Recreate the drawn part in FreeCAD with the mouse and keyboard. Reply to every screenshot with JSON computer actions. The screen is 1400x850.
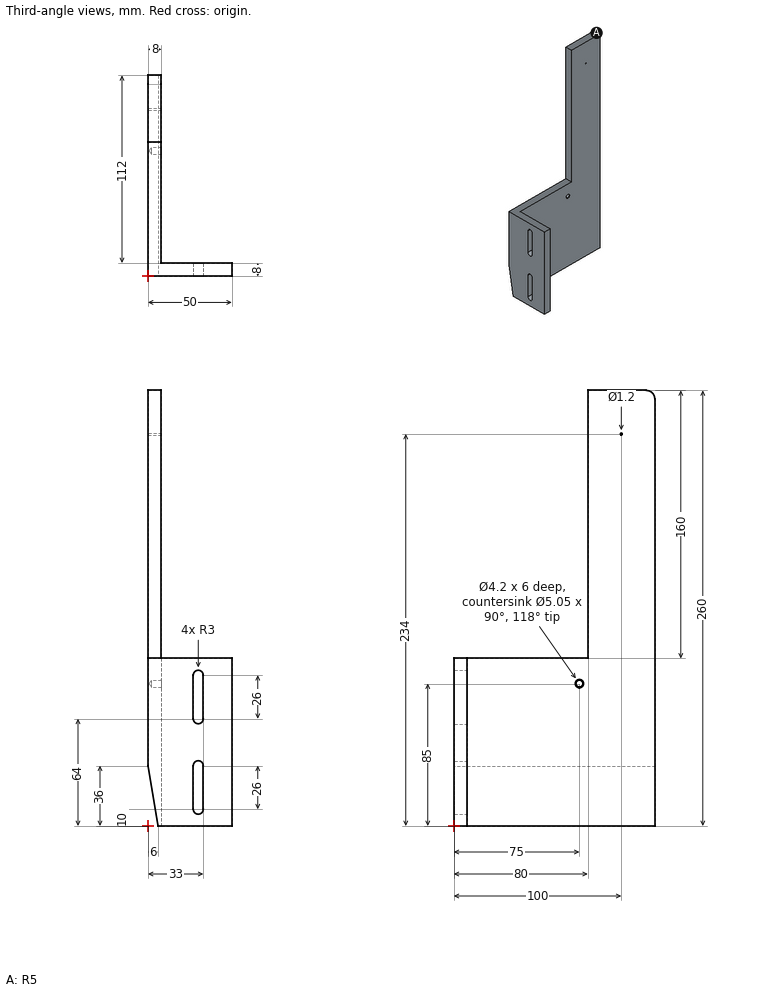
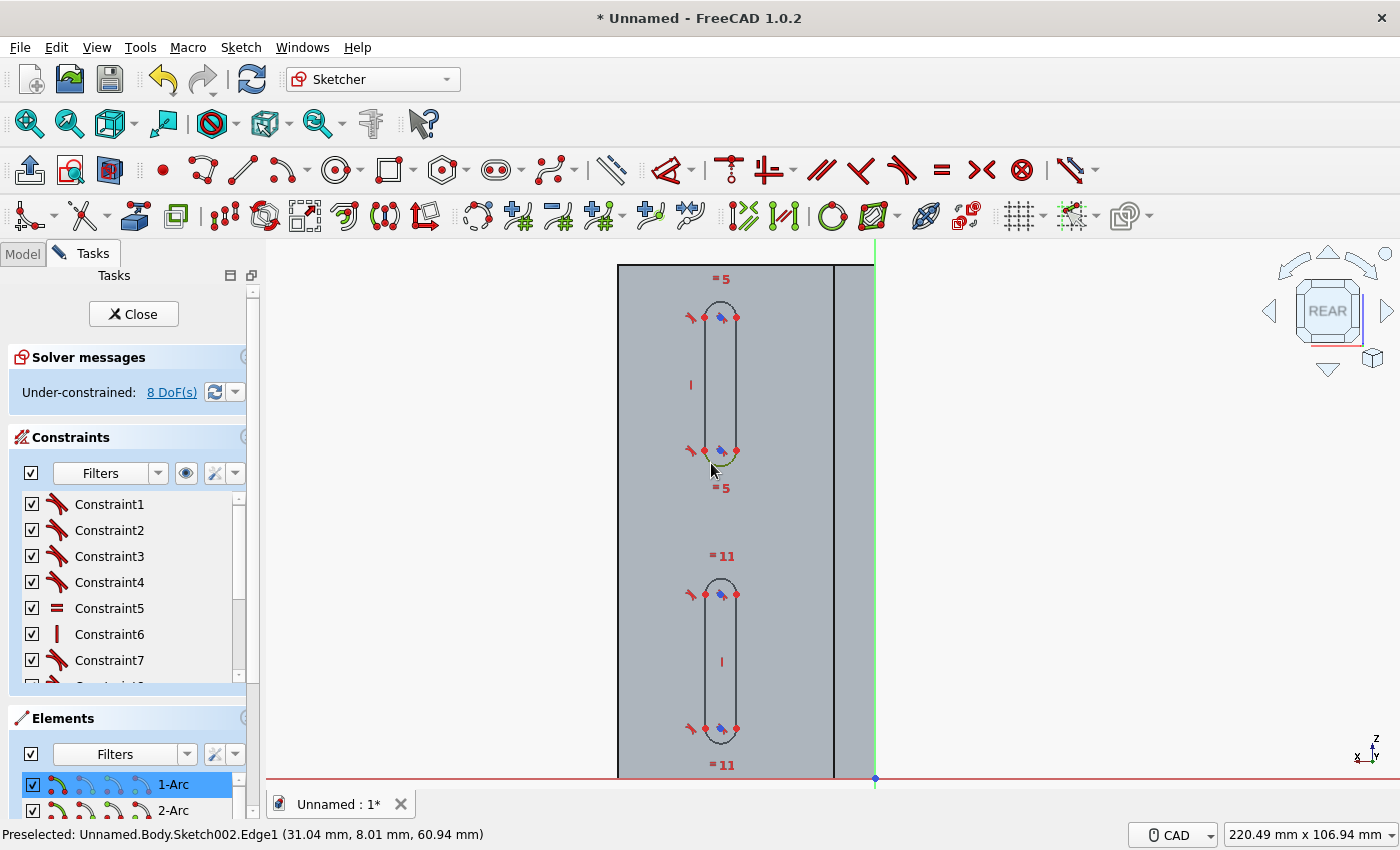
{"action": "left_click", "coordinate": [712, 741]}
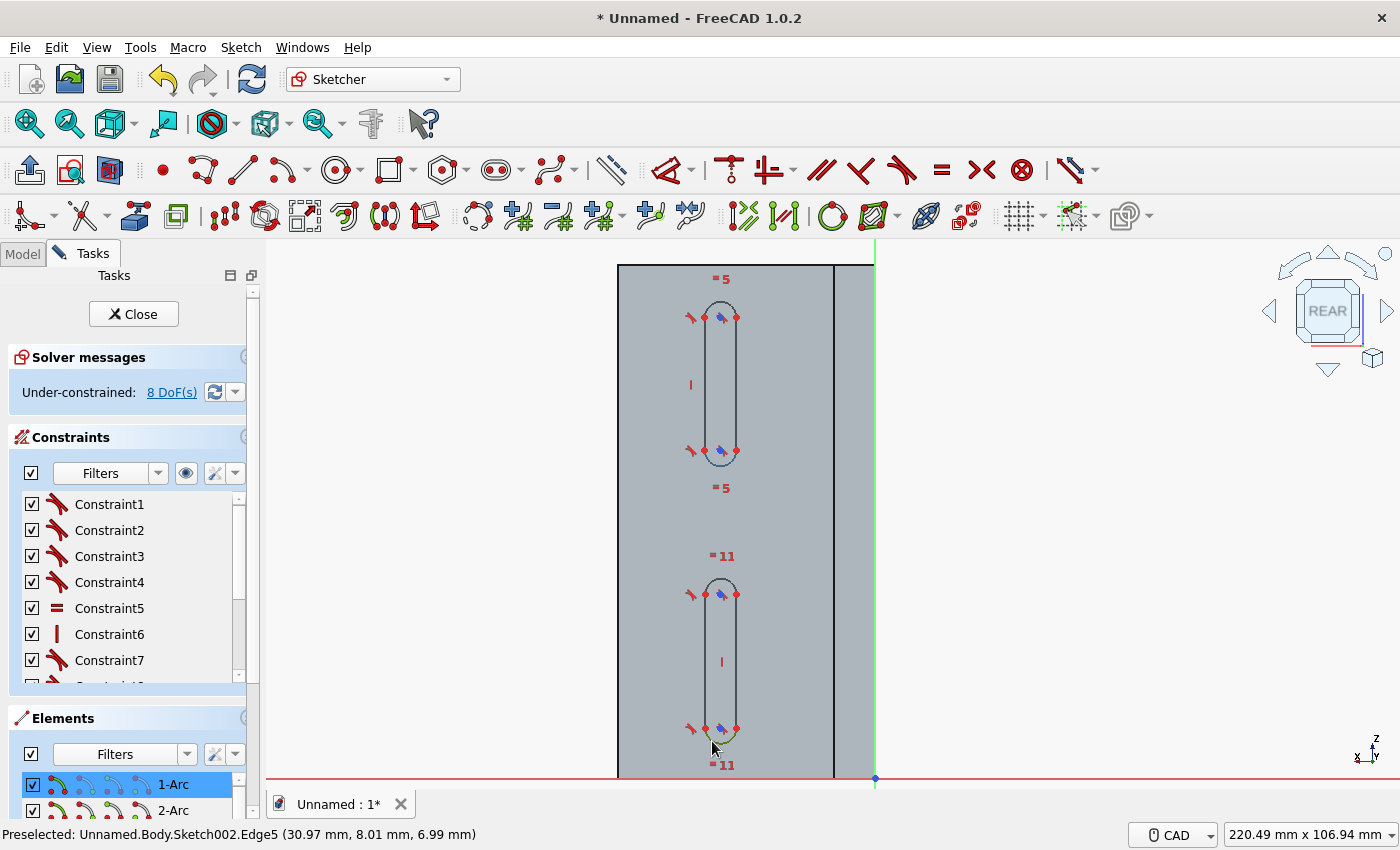
{"action": "left_click", "coordinate": [942, 170]}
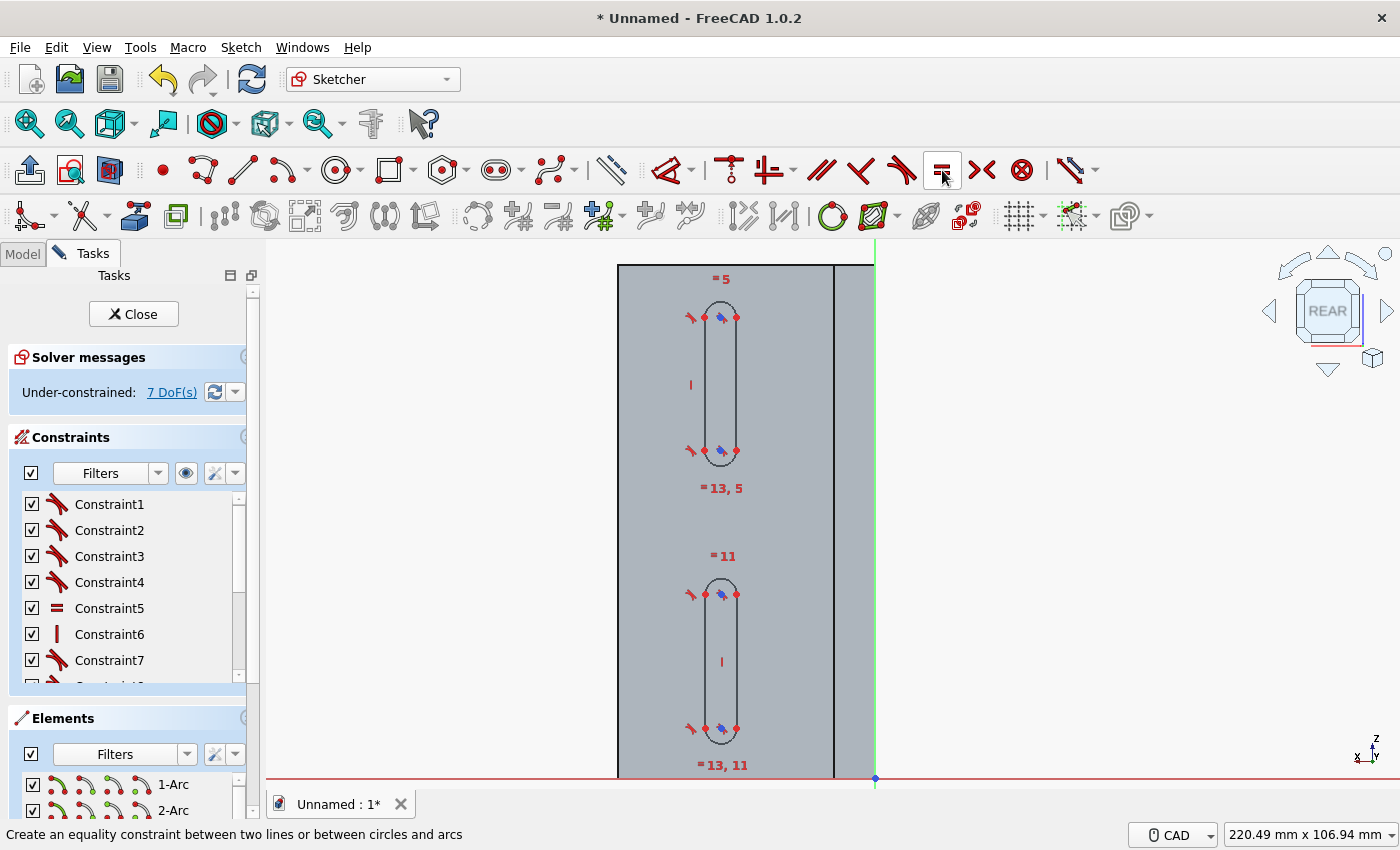
{"action": "left_click", "coordinate": [666, 170]}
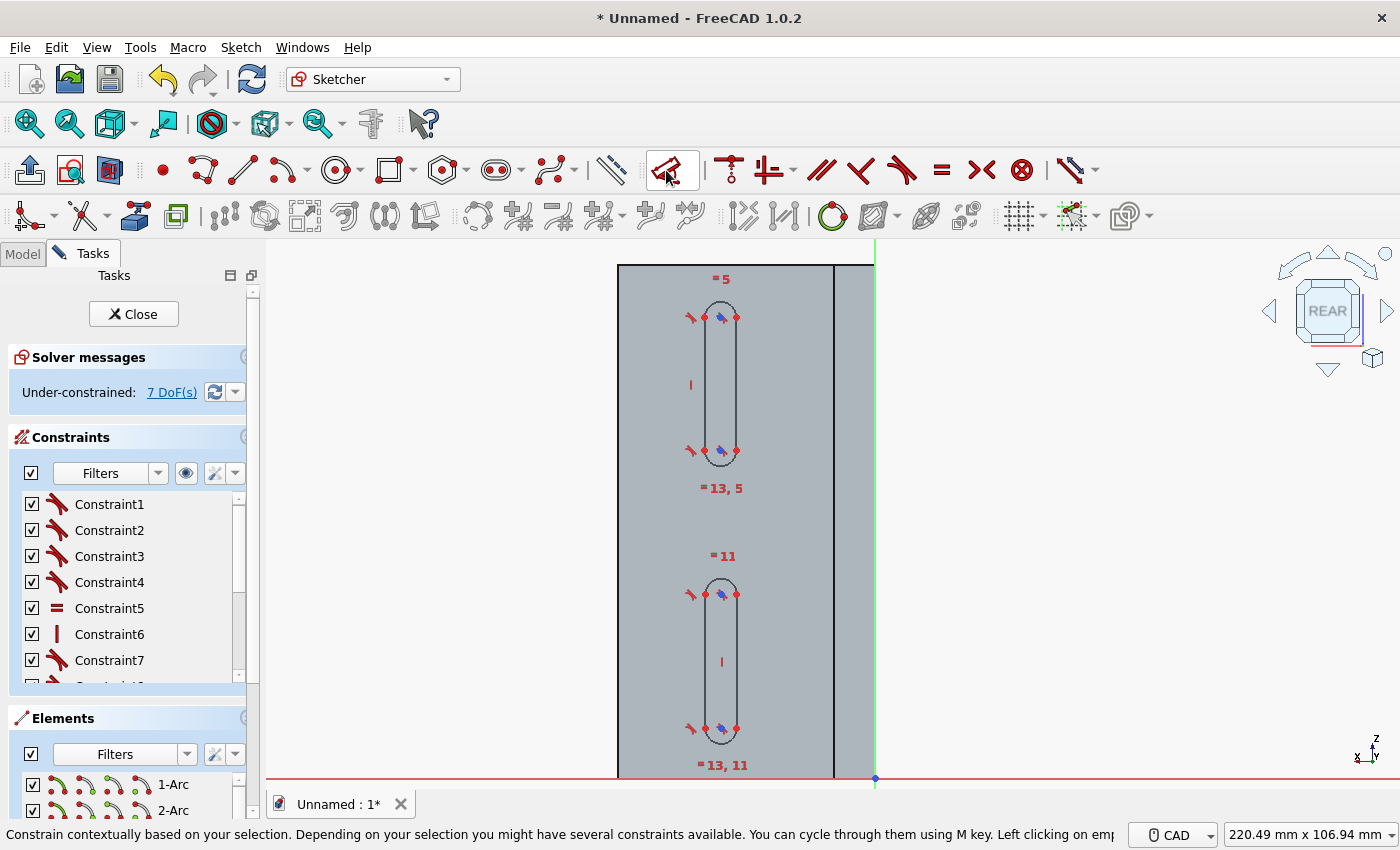
{"action": "scroll", "coordinate": [711, 463], "scroll_direction": "up", "scroll_amount": 5}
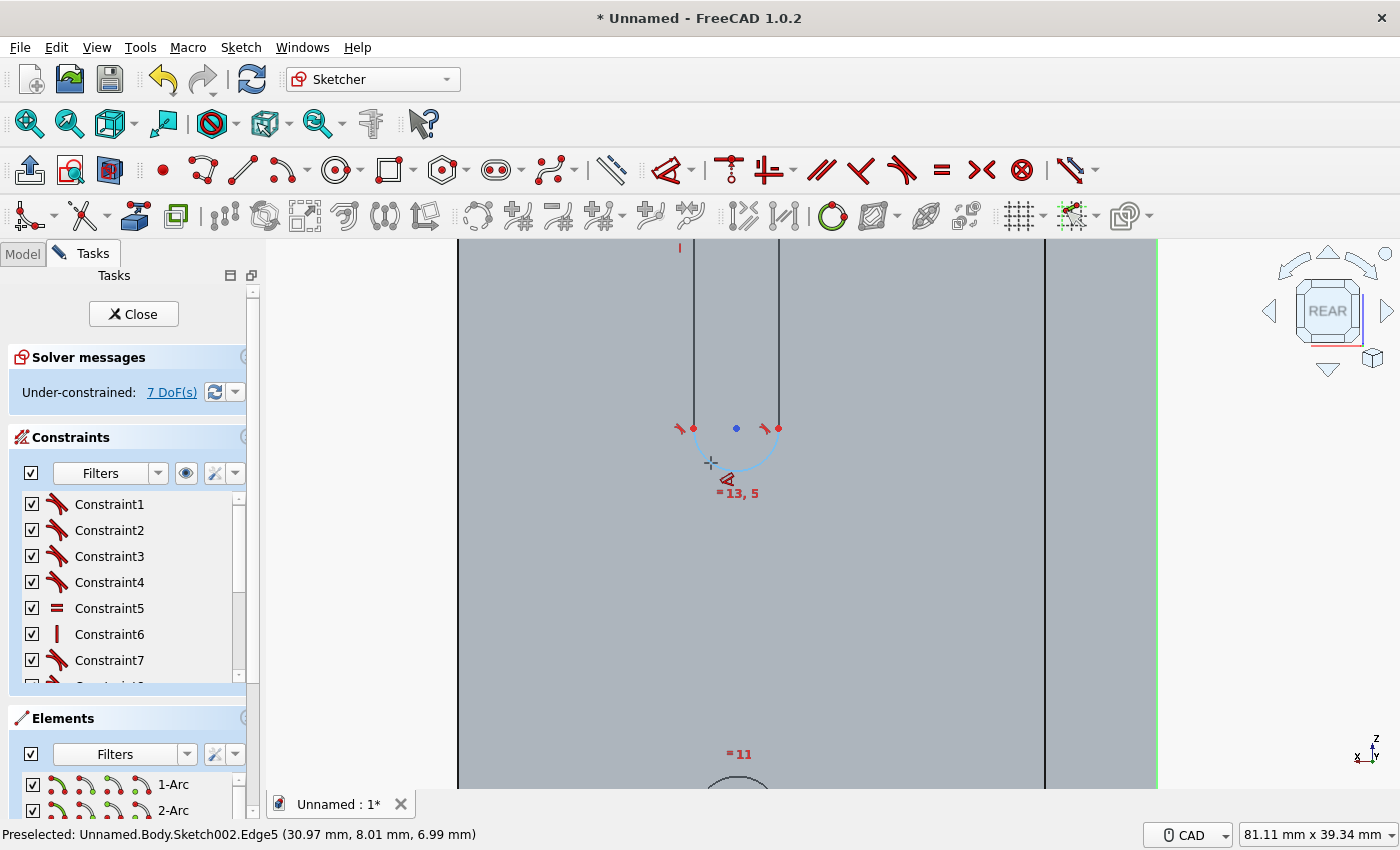
{"action": "left_click", "coordinate": [711, 463]}
{"action": "left_click", "coordinate": [692, 489]}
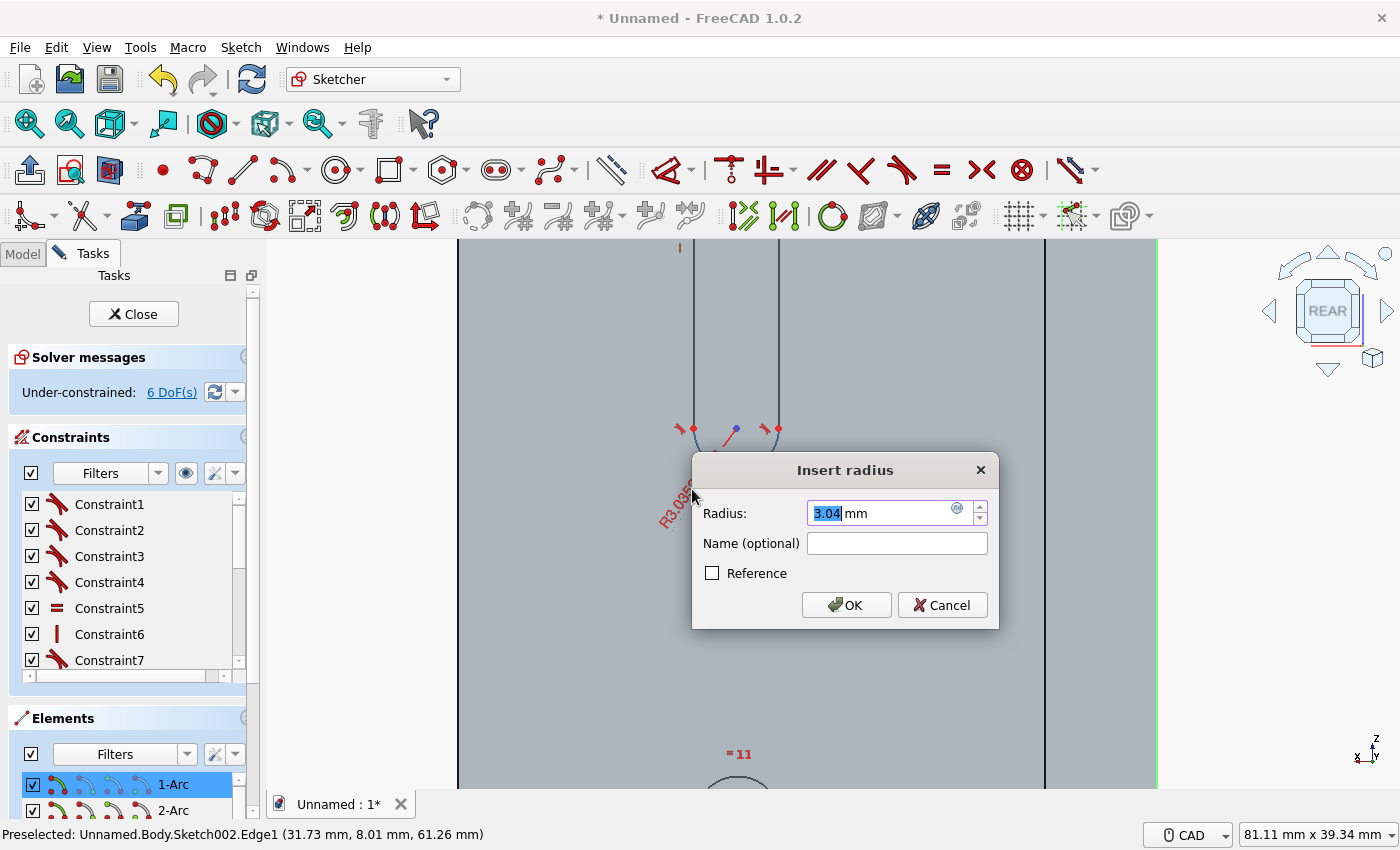
{"action": "type", "text": "3"}
{"action": "key", "text": "Return"}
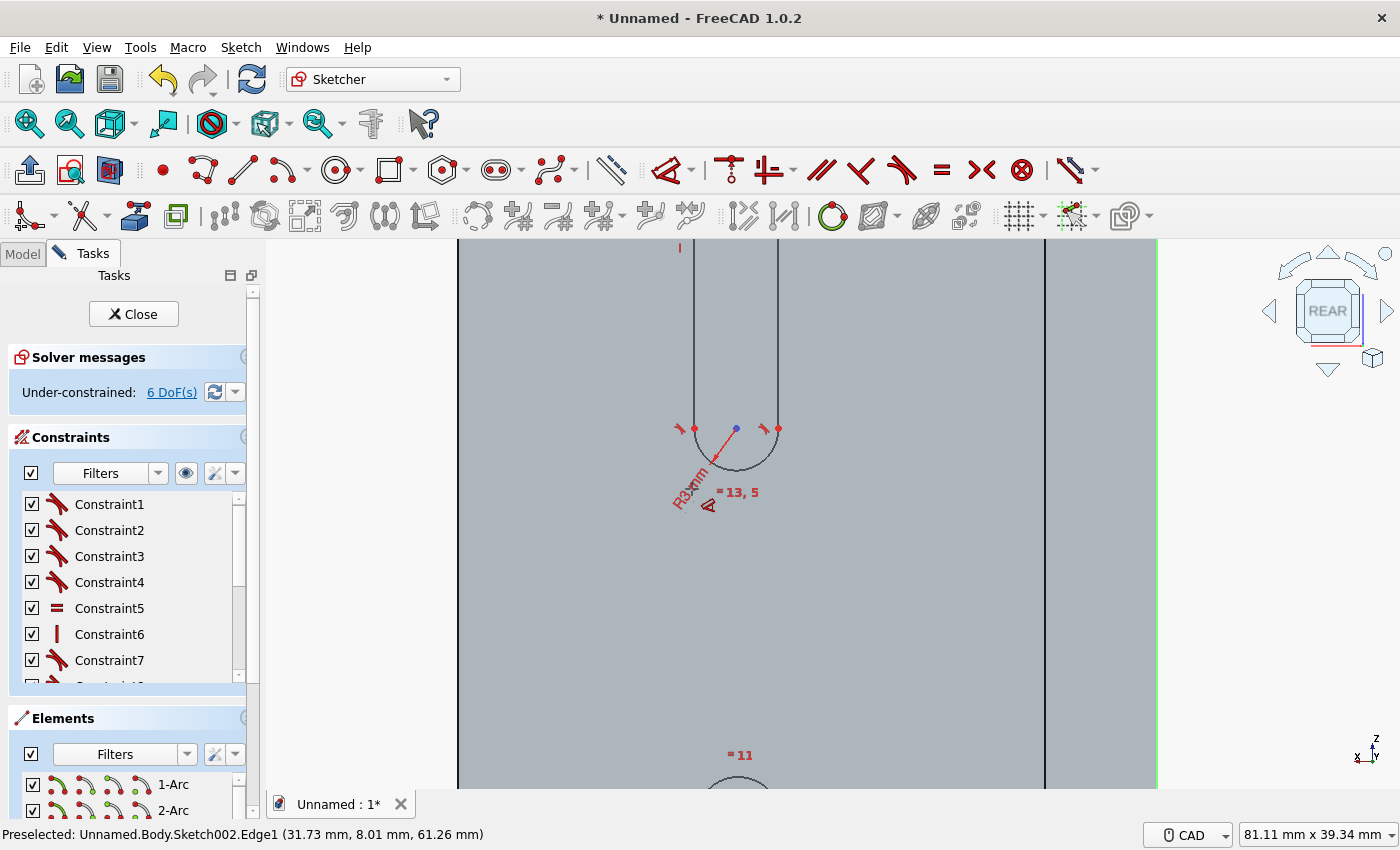
{"action": "scroll", "coordinate": [711, 463], "scroll_direction": "down", "scroll_amount": 7}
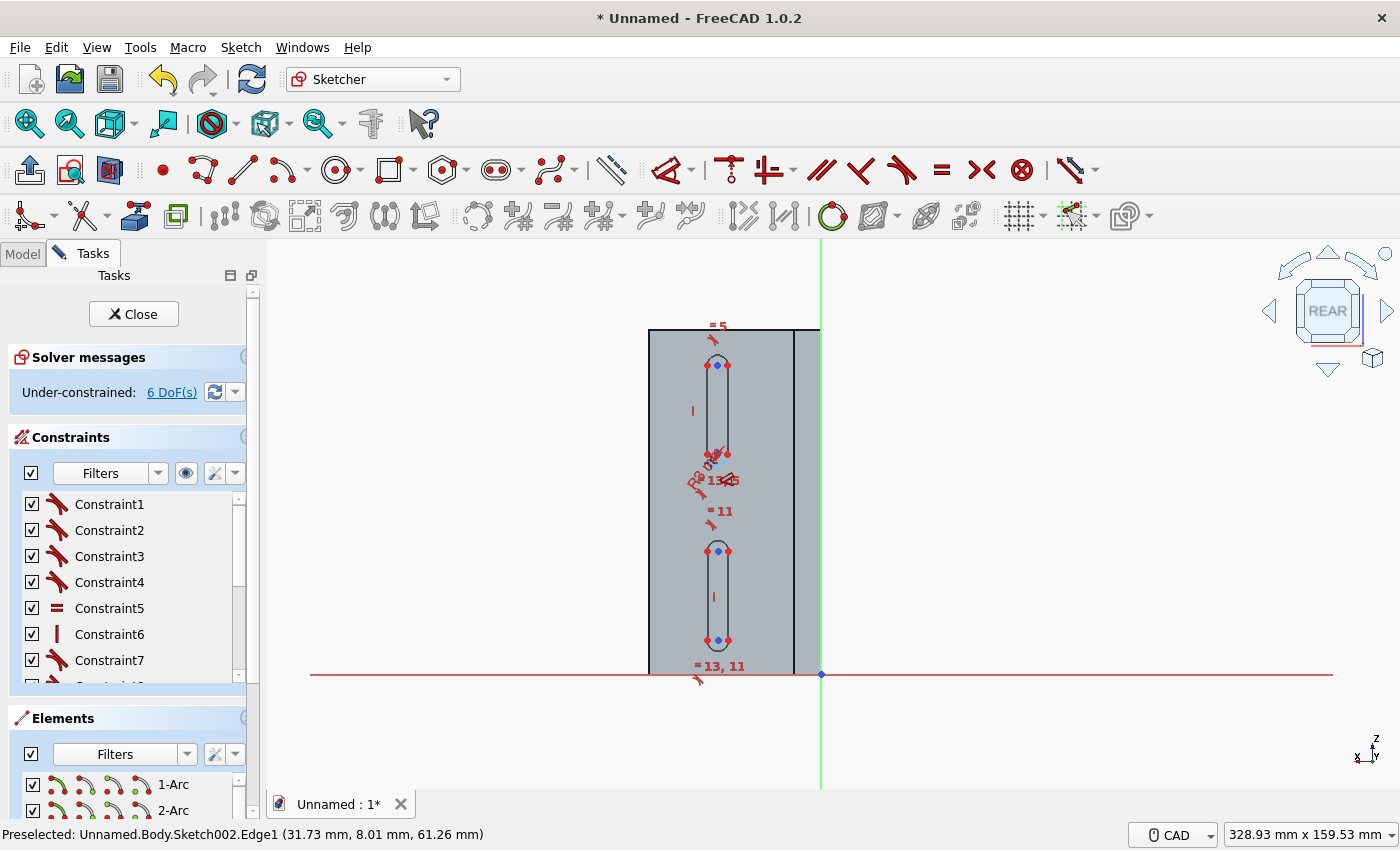
{"action": "left_click", "coordinate": [707, 428]}
{"action": "left_click", "coordinate": [673, 410]}